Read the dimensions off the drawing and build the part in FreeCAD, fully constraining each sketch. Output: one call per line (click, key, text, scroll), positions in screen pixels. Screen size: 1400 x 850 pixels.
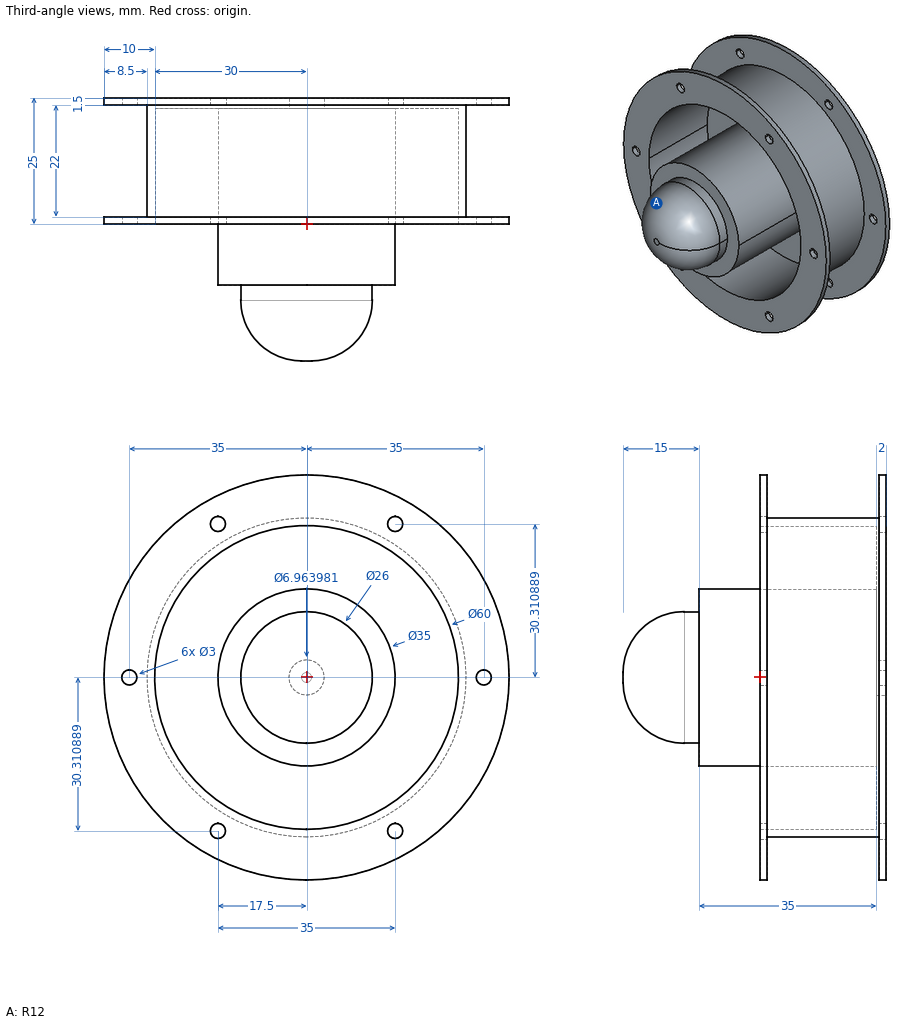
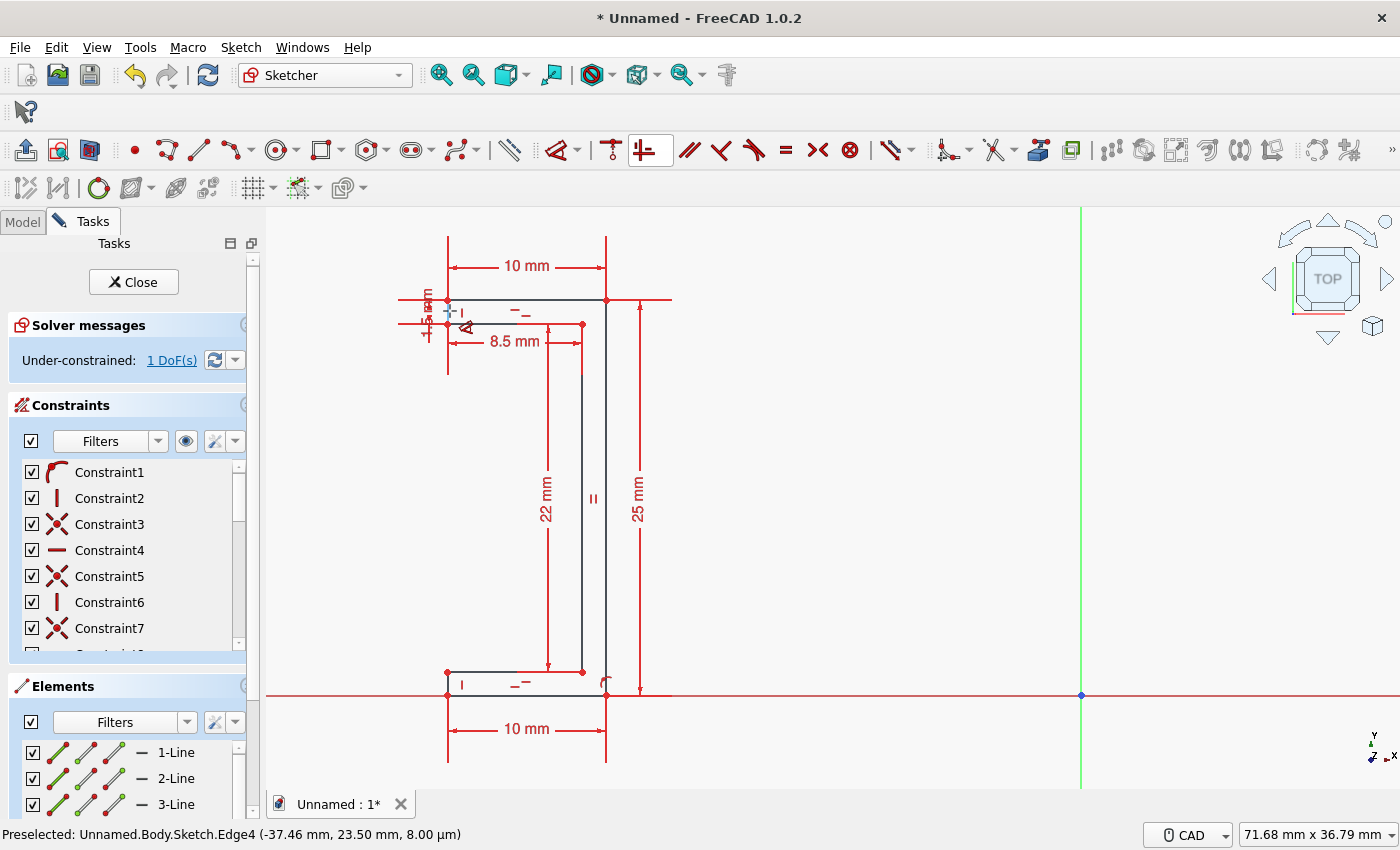
click(606, 696)
click(844, 730)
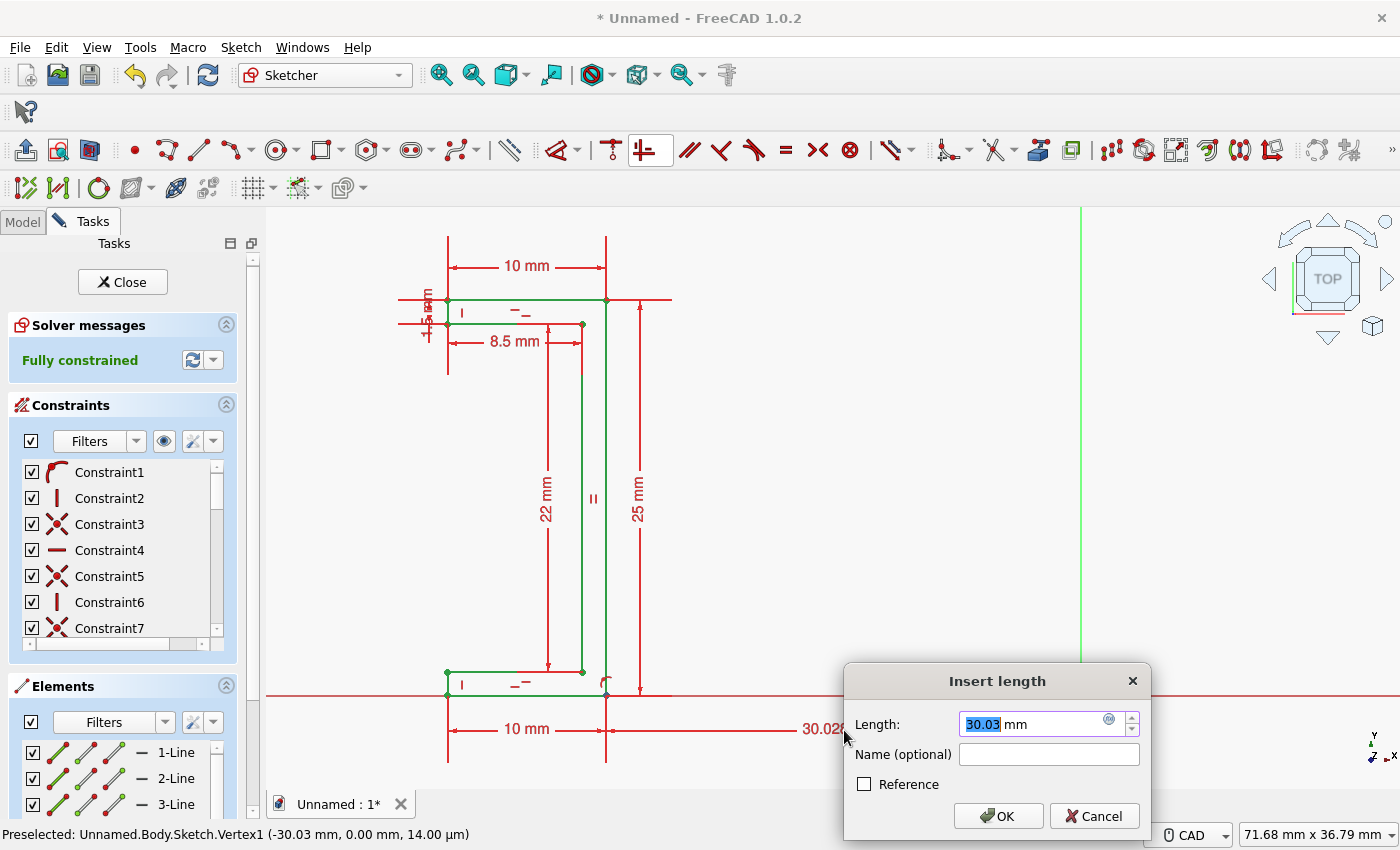
text(30)
key(Return)
key(Escape)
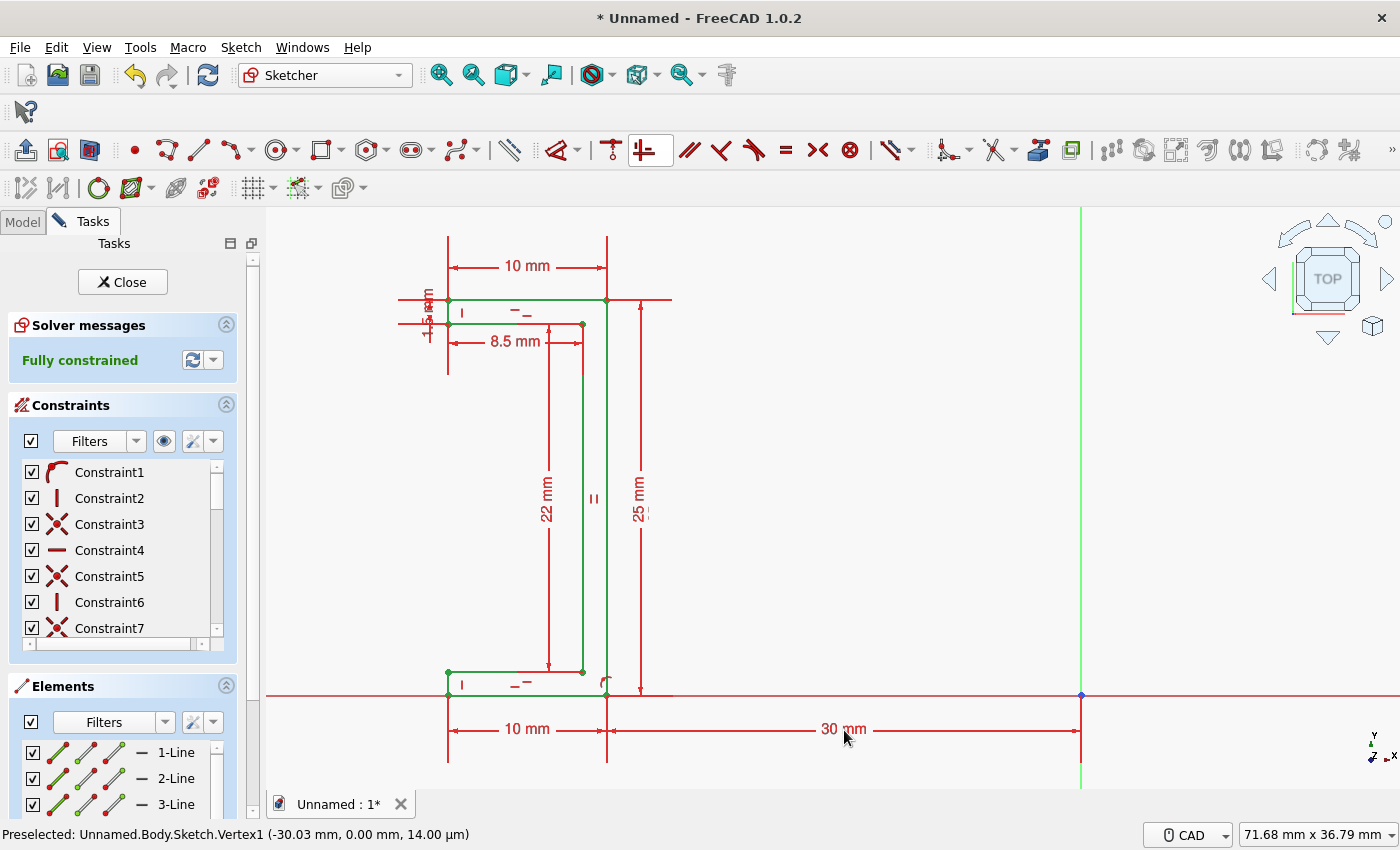
click(123, 282)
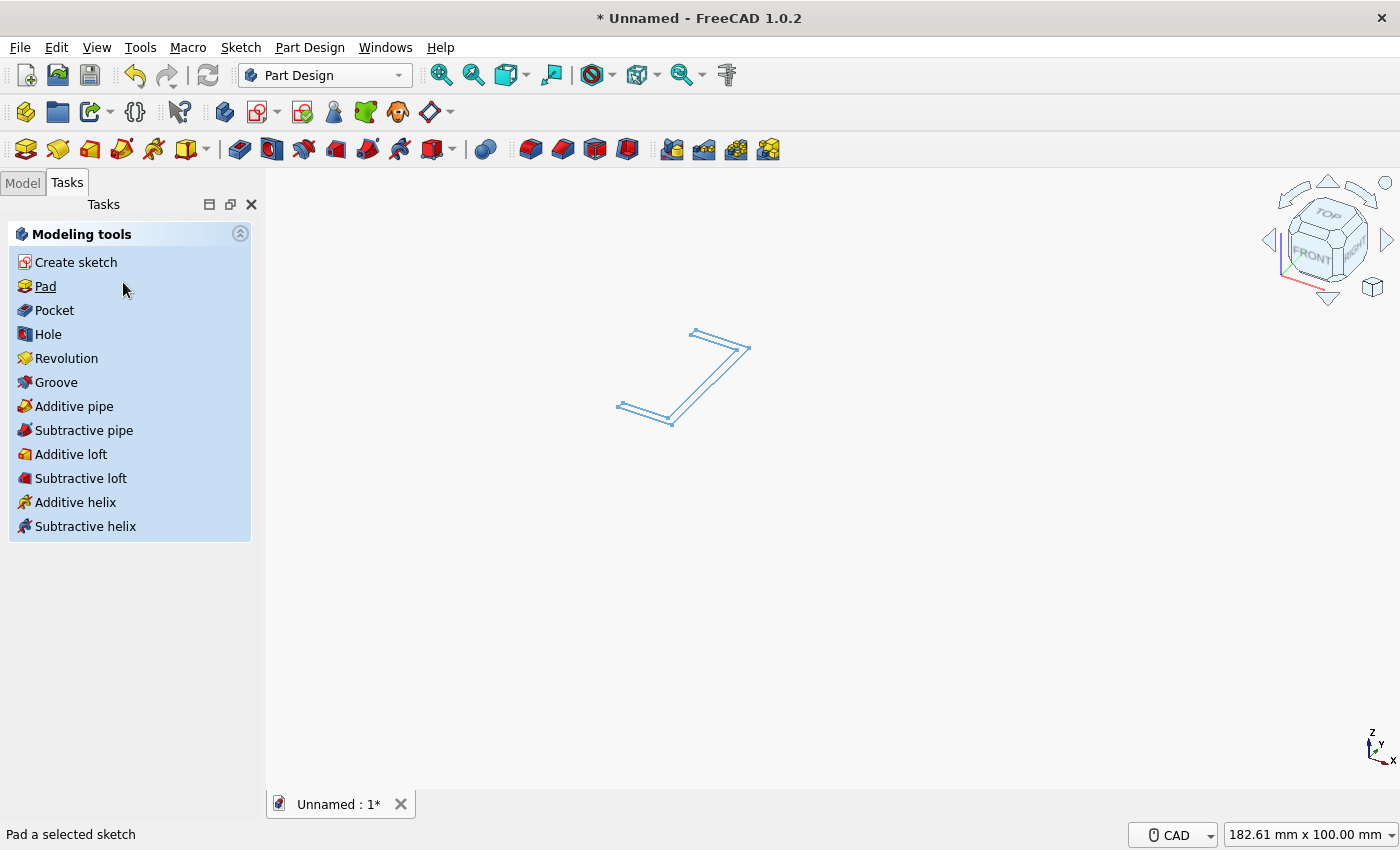
click(58, 150)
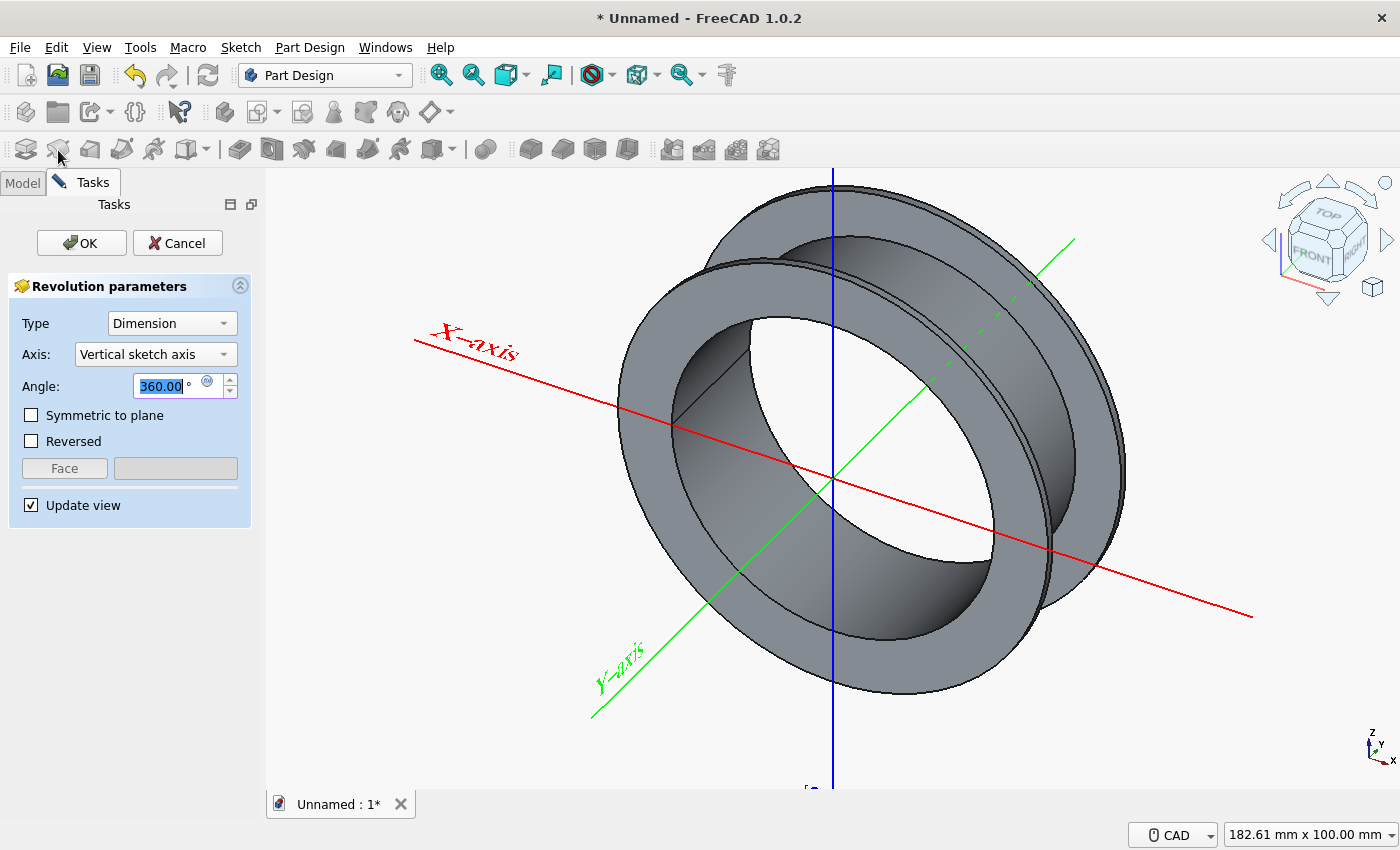
click(82, 243)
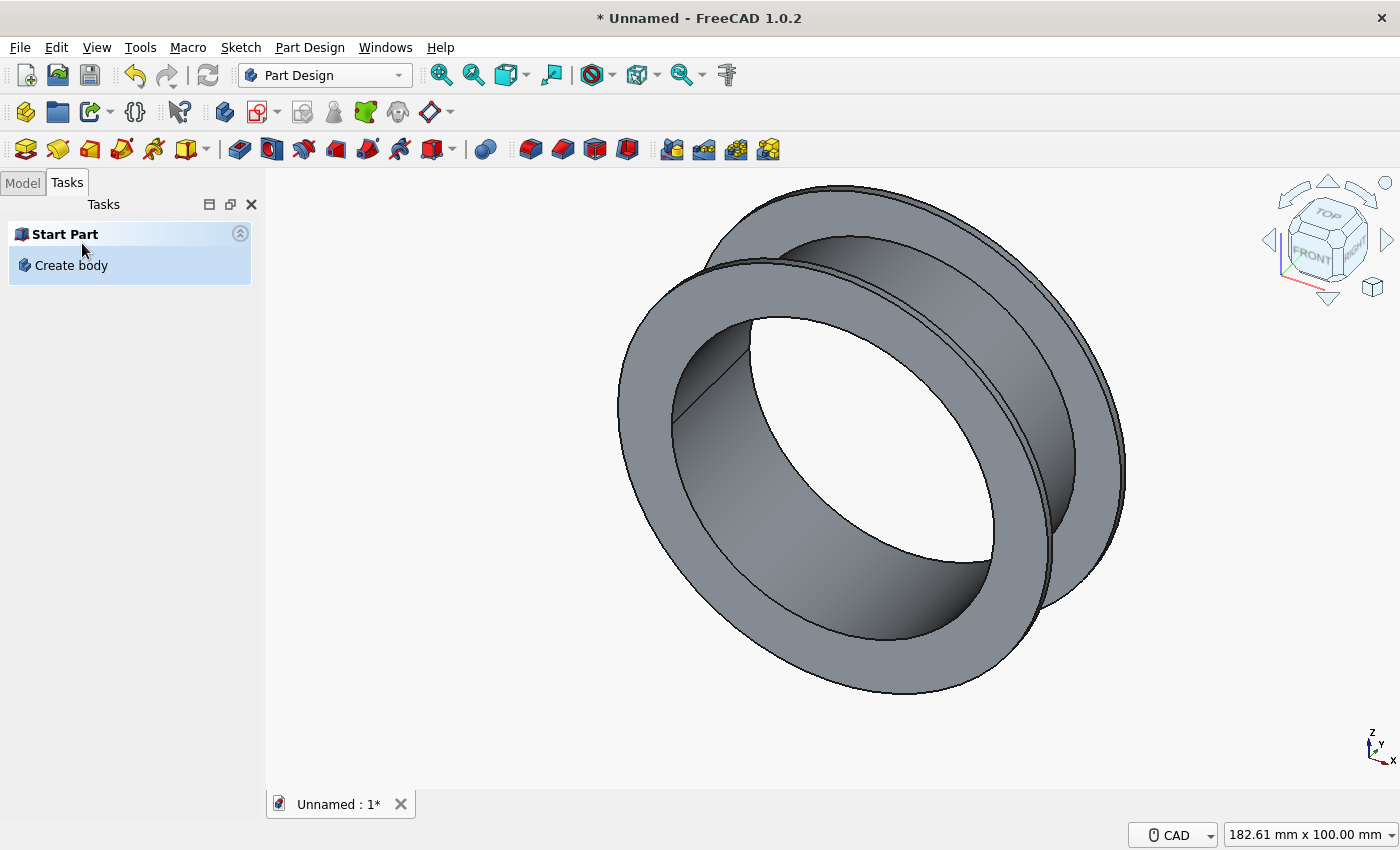
click(442, 76)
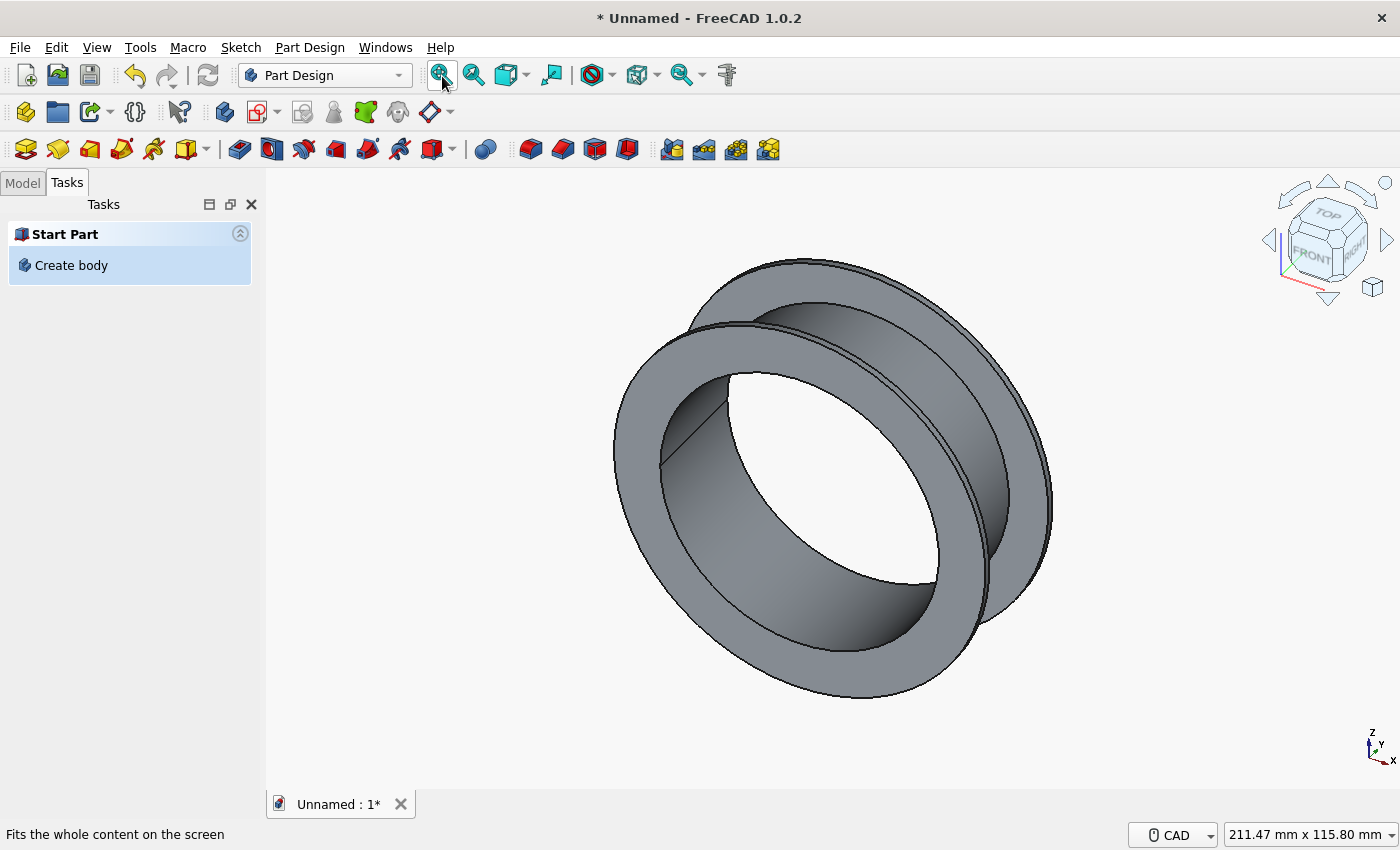
key(4)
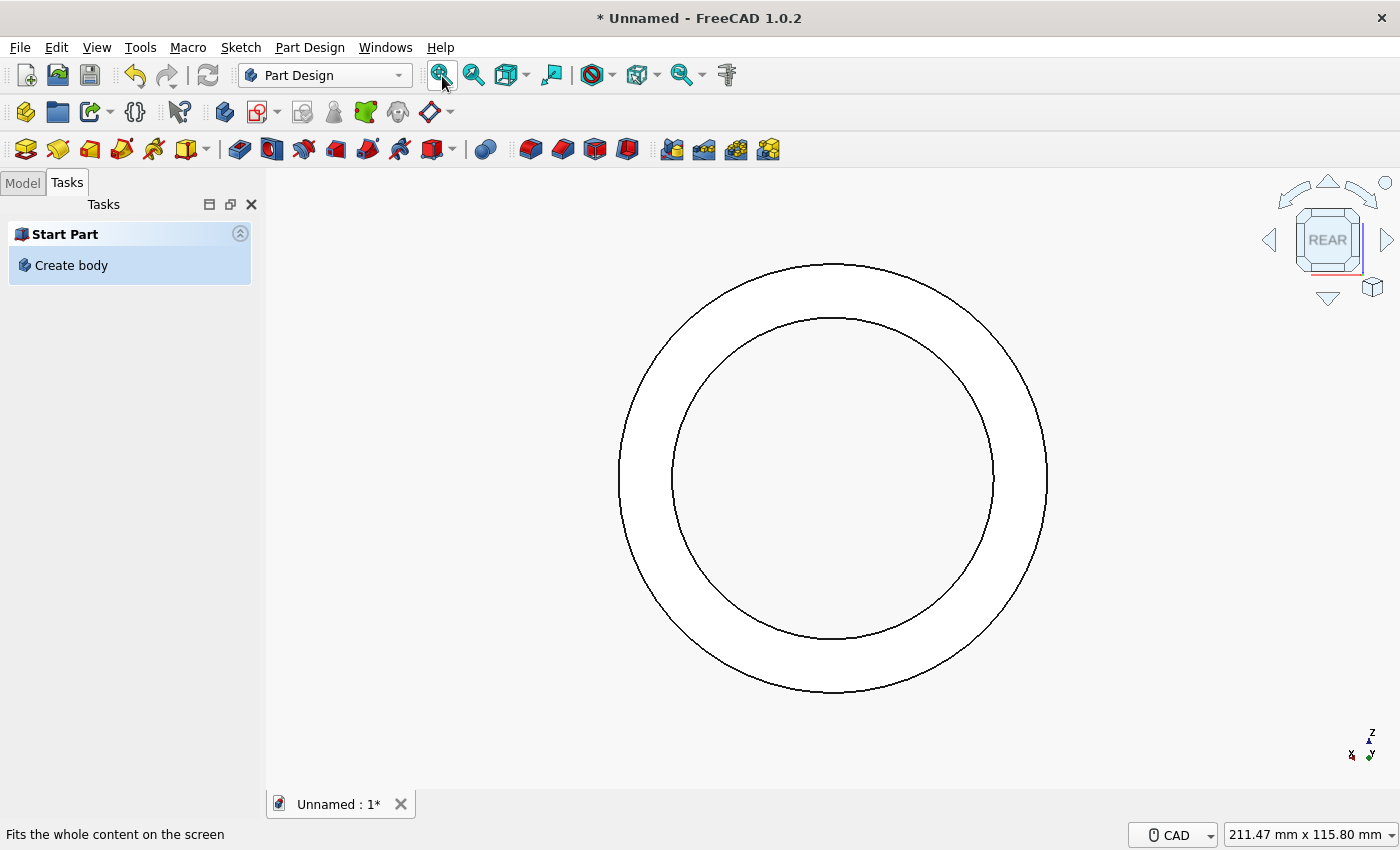
click(649, 477)